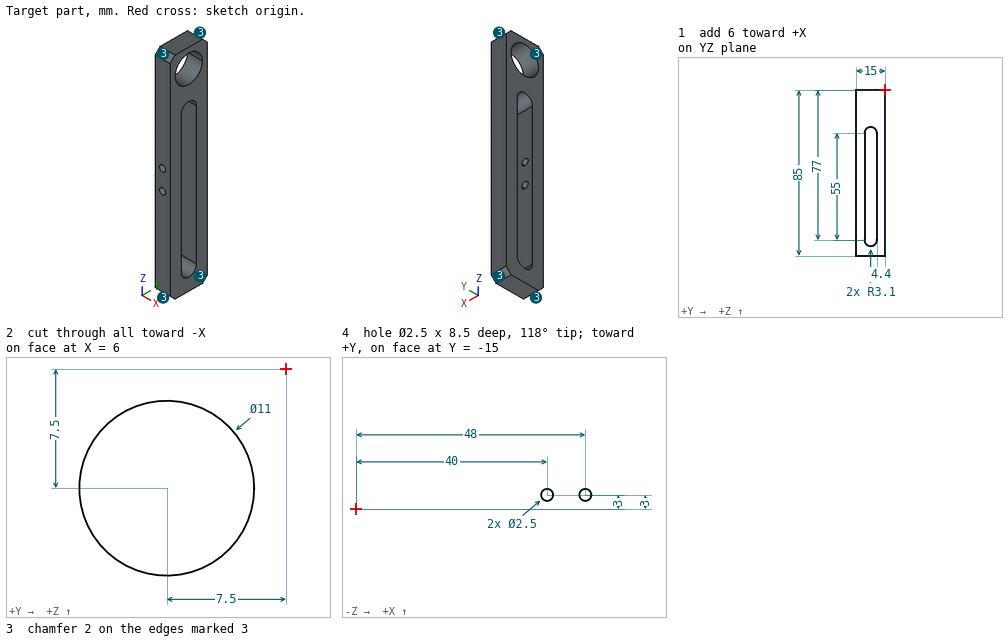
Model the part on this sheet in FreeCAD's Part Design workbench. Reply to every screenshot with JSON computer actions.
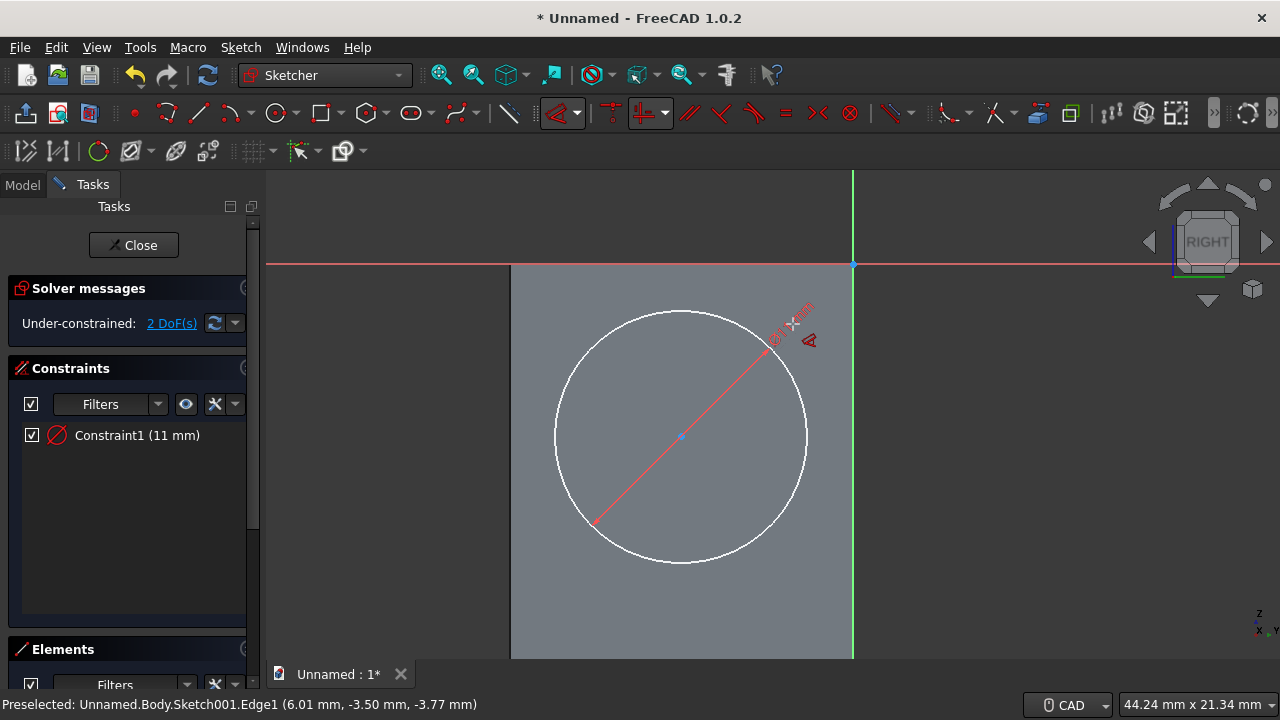
{"action": "left_click", "coordinate": [681, 437]}
{"action": "left_click", "coordinate": [767, 230]}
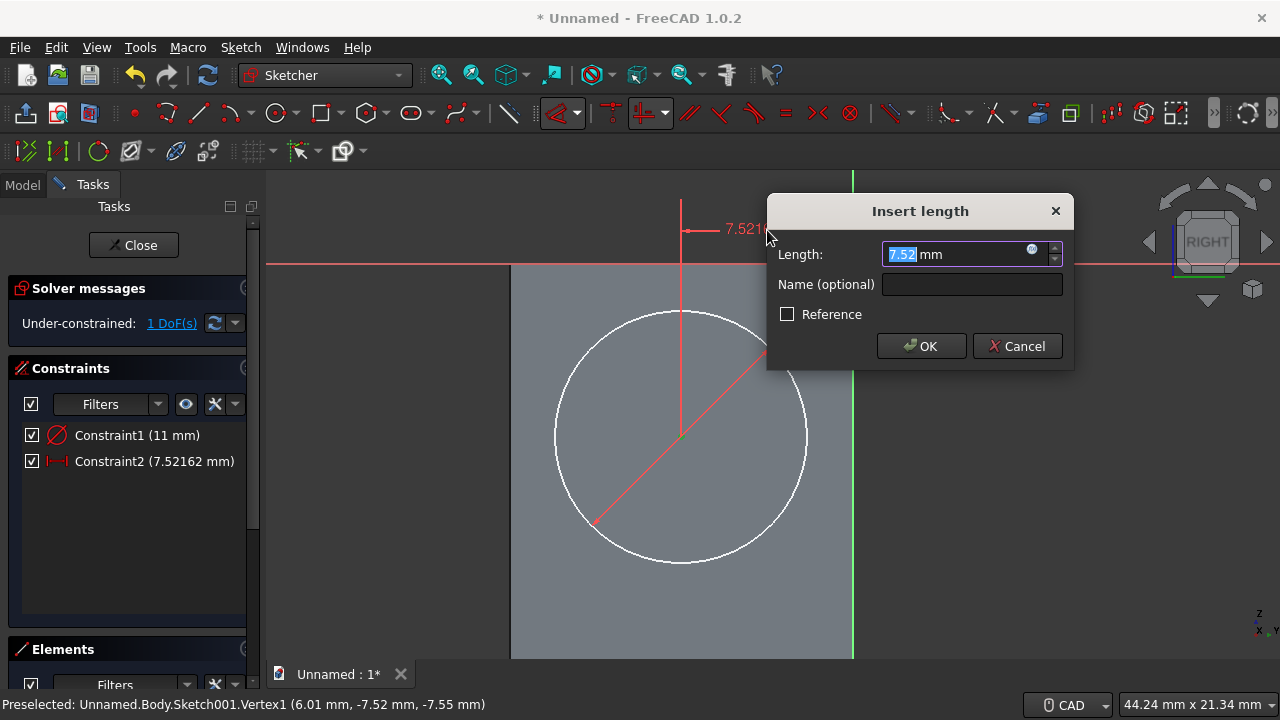
{"action": "type", "text": "7.5"}
{"action": "key", "text": "Return"}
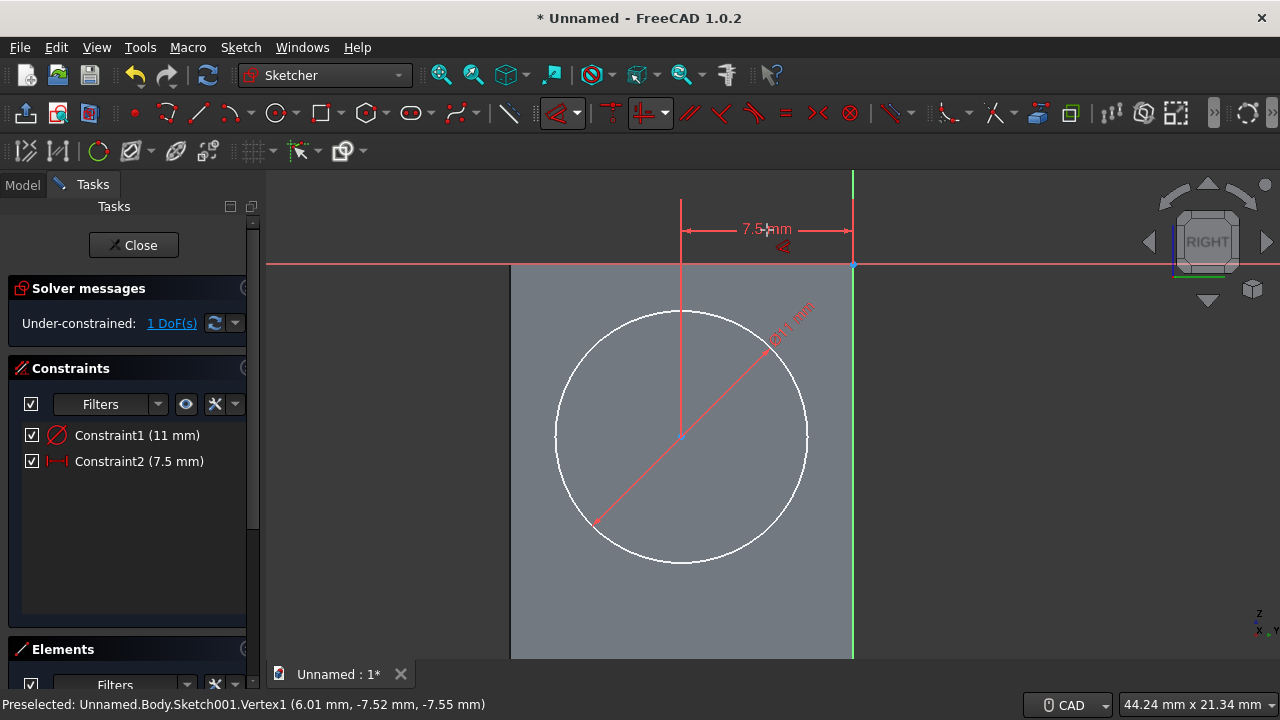
{"action": "left_click", "coordinate": [681, 437]}
{"action": "left_click", "coordinate": [887, 351]}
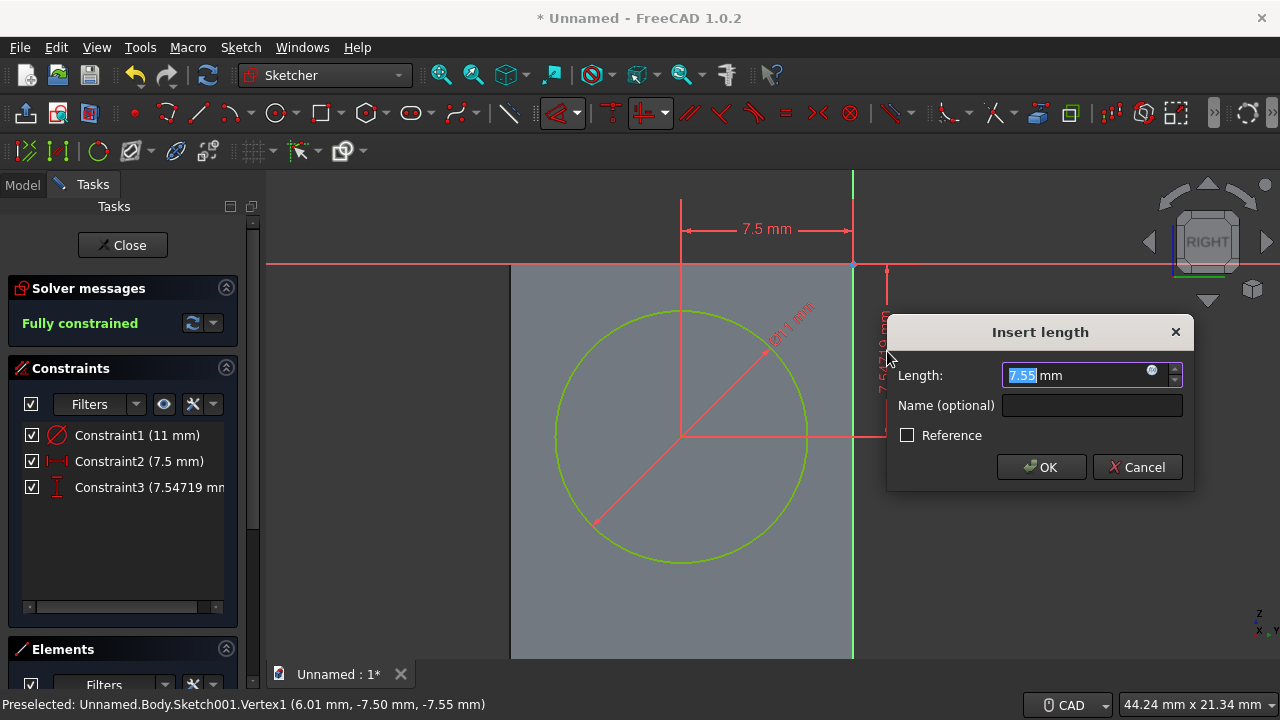
{"action": "type", "text": "7.5"}
{"action": "key", "text": "Return"}
{"action": "key", "text": "Escape"}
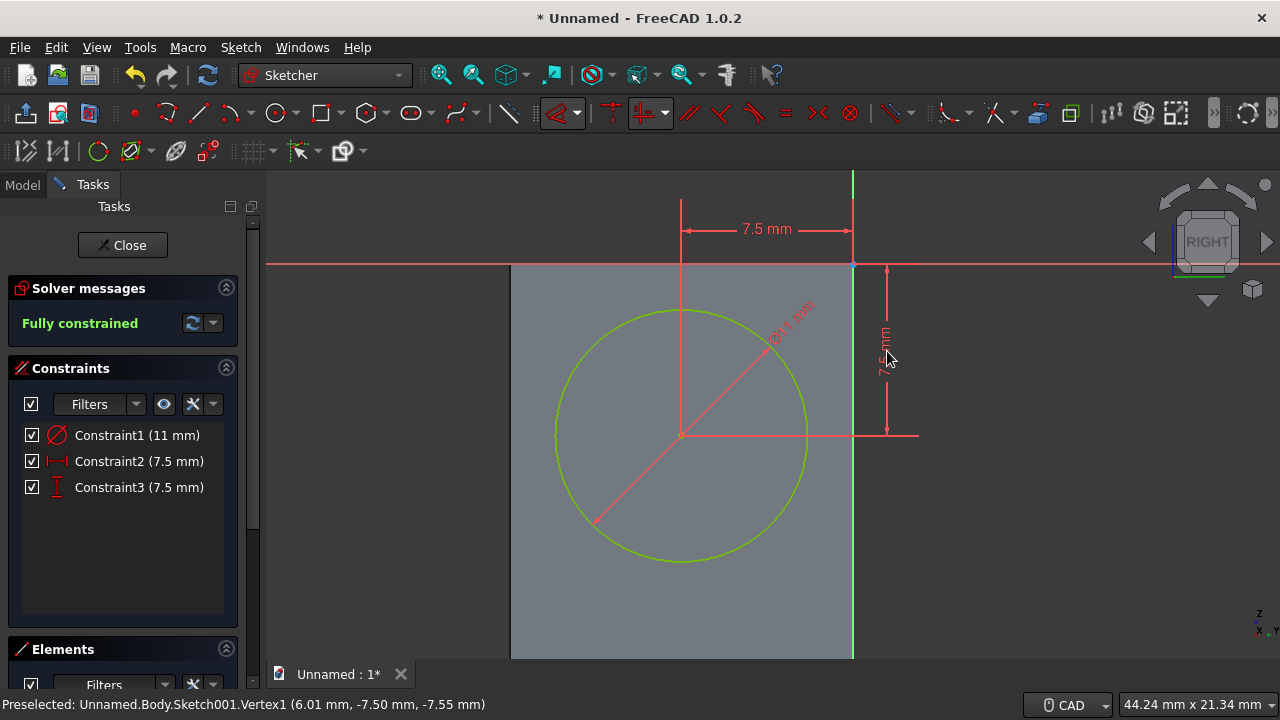
{"action": "left_click", "coordinate": [123, 245]}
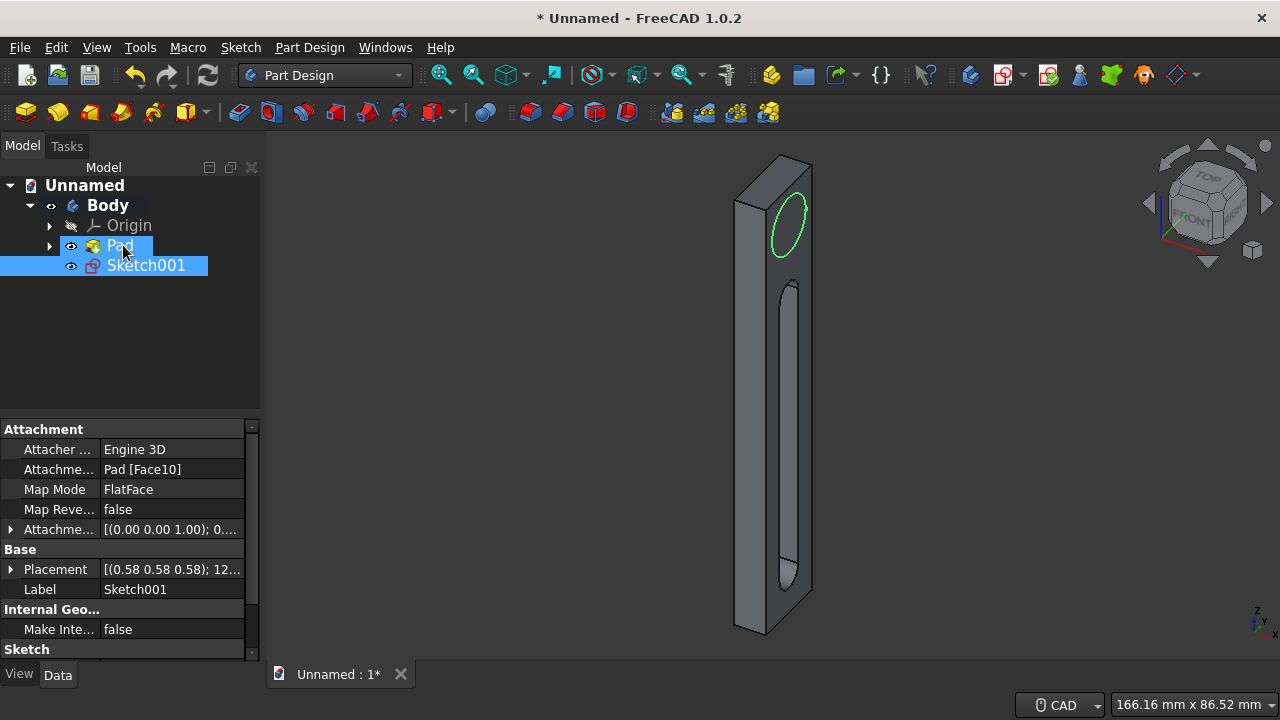
{"action": "left_click", "coordinate": [240, 112]}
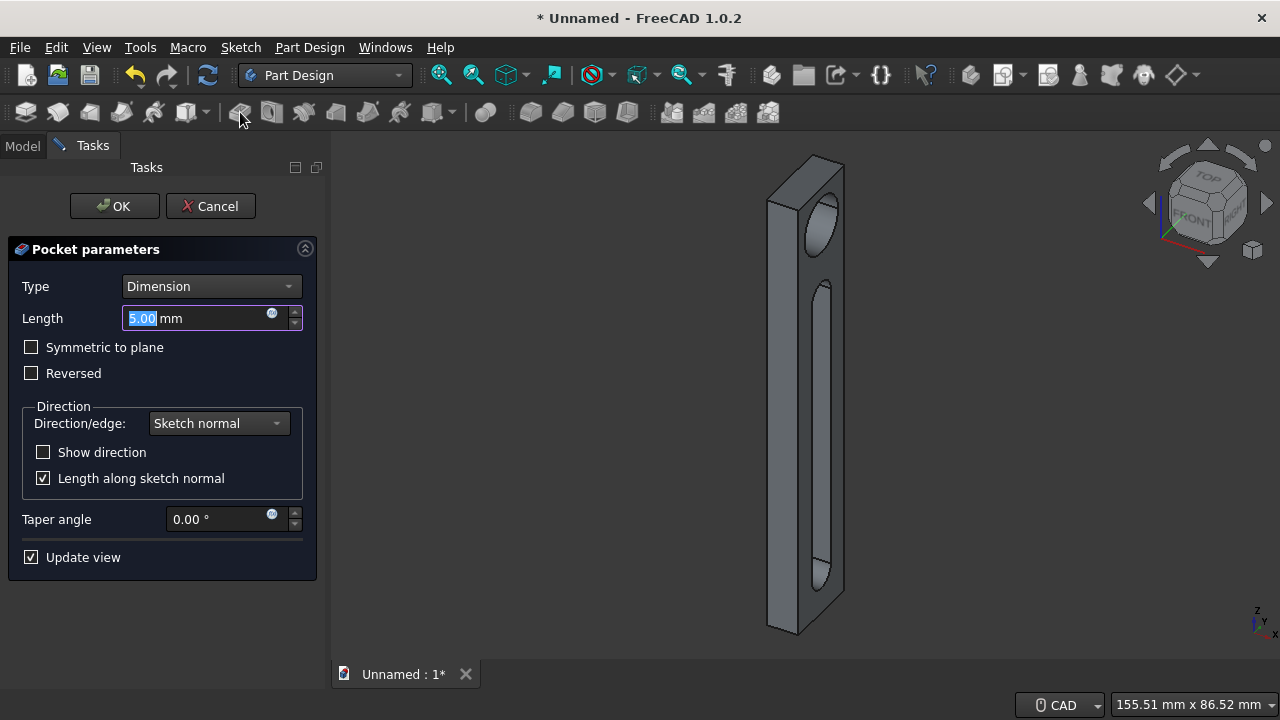
{"action": "left_click", "coordinate": [212, 286]}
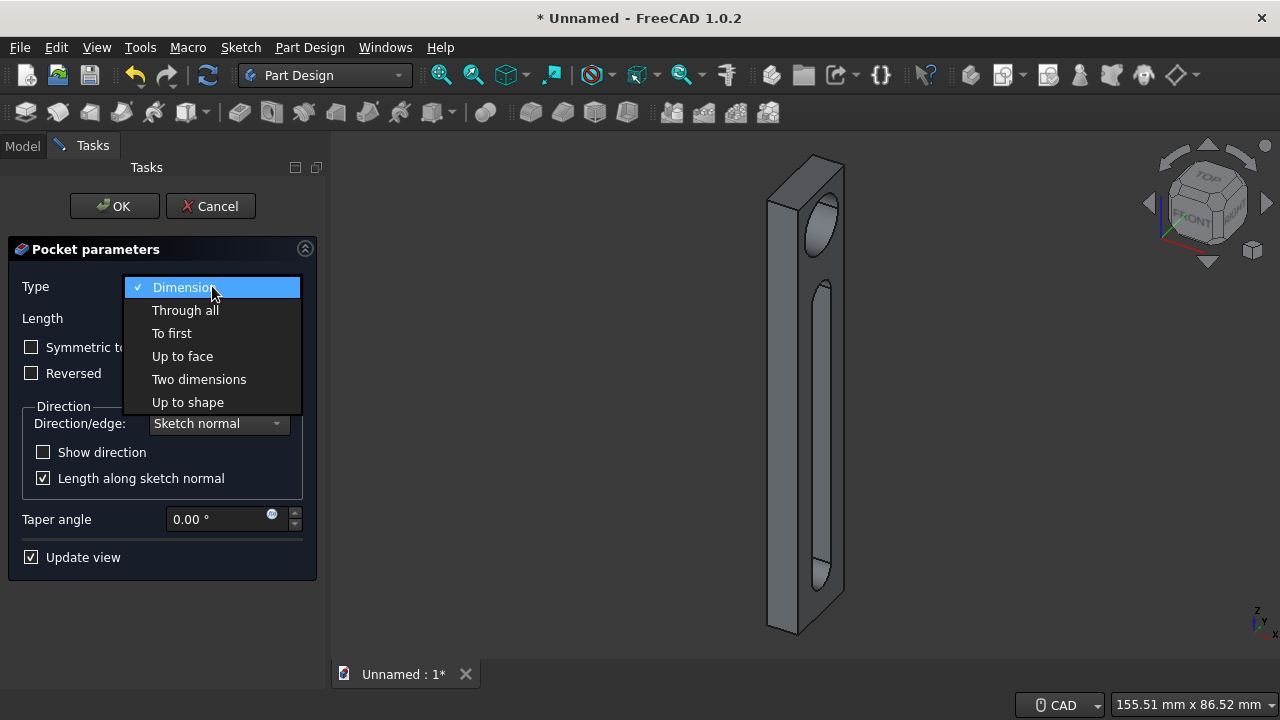
{"action": "left_click", "coordinate": [212, 310]}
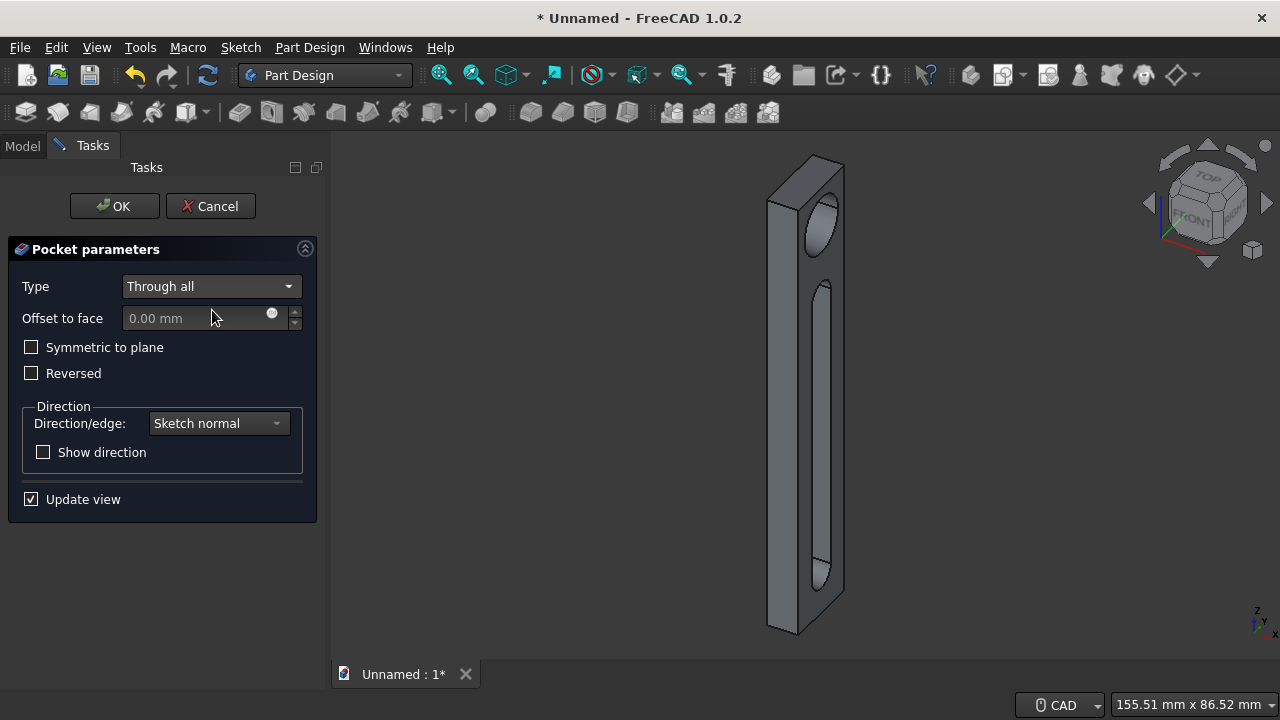
{"action": "left_click", "coordinate": [115, 206]}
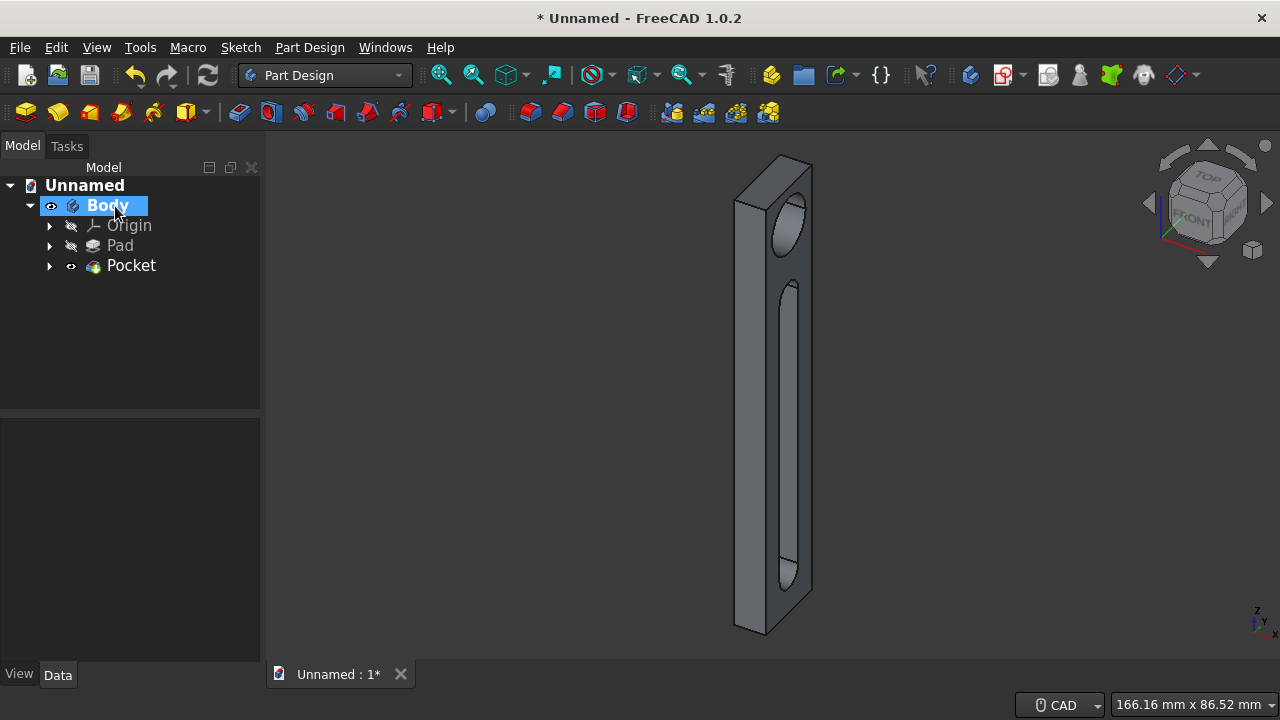
{"action": "left_click", "coordinate": [750, 204]}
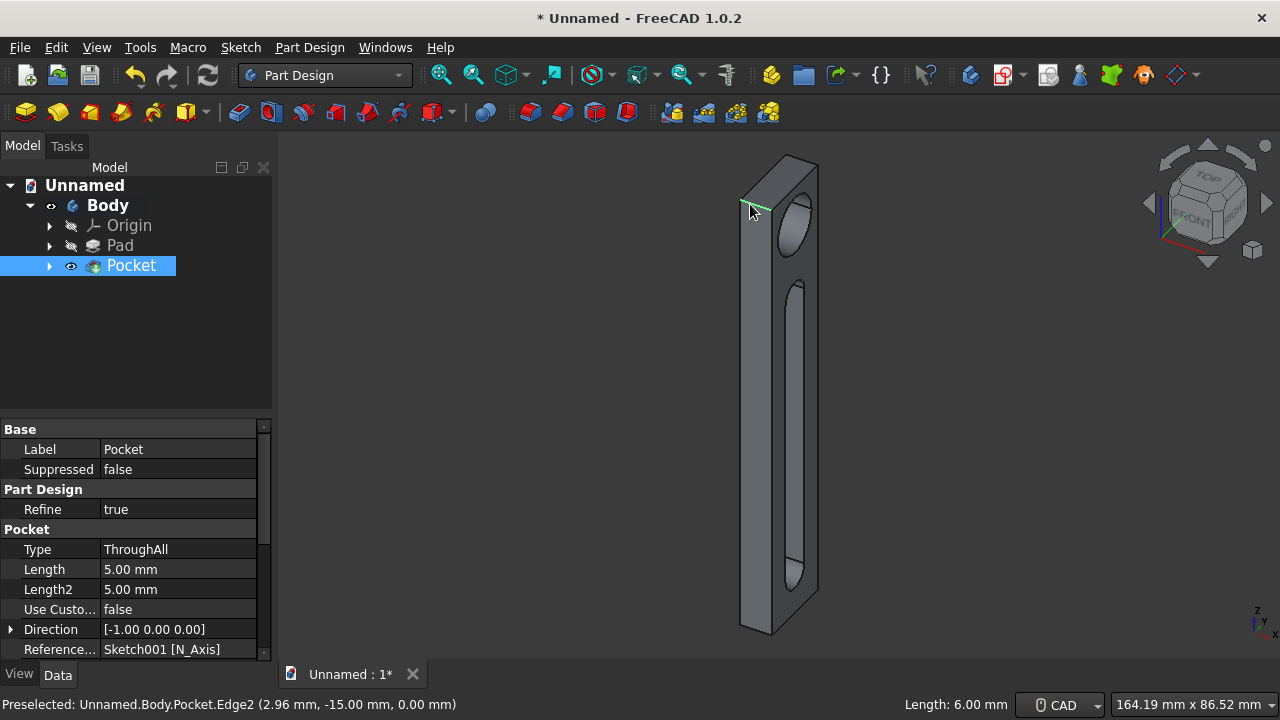
{"action": "key", "text": "0"}